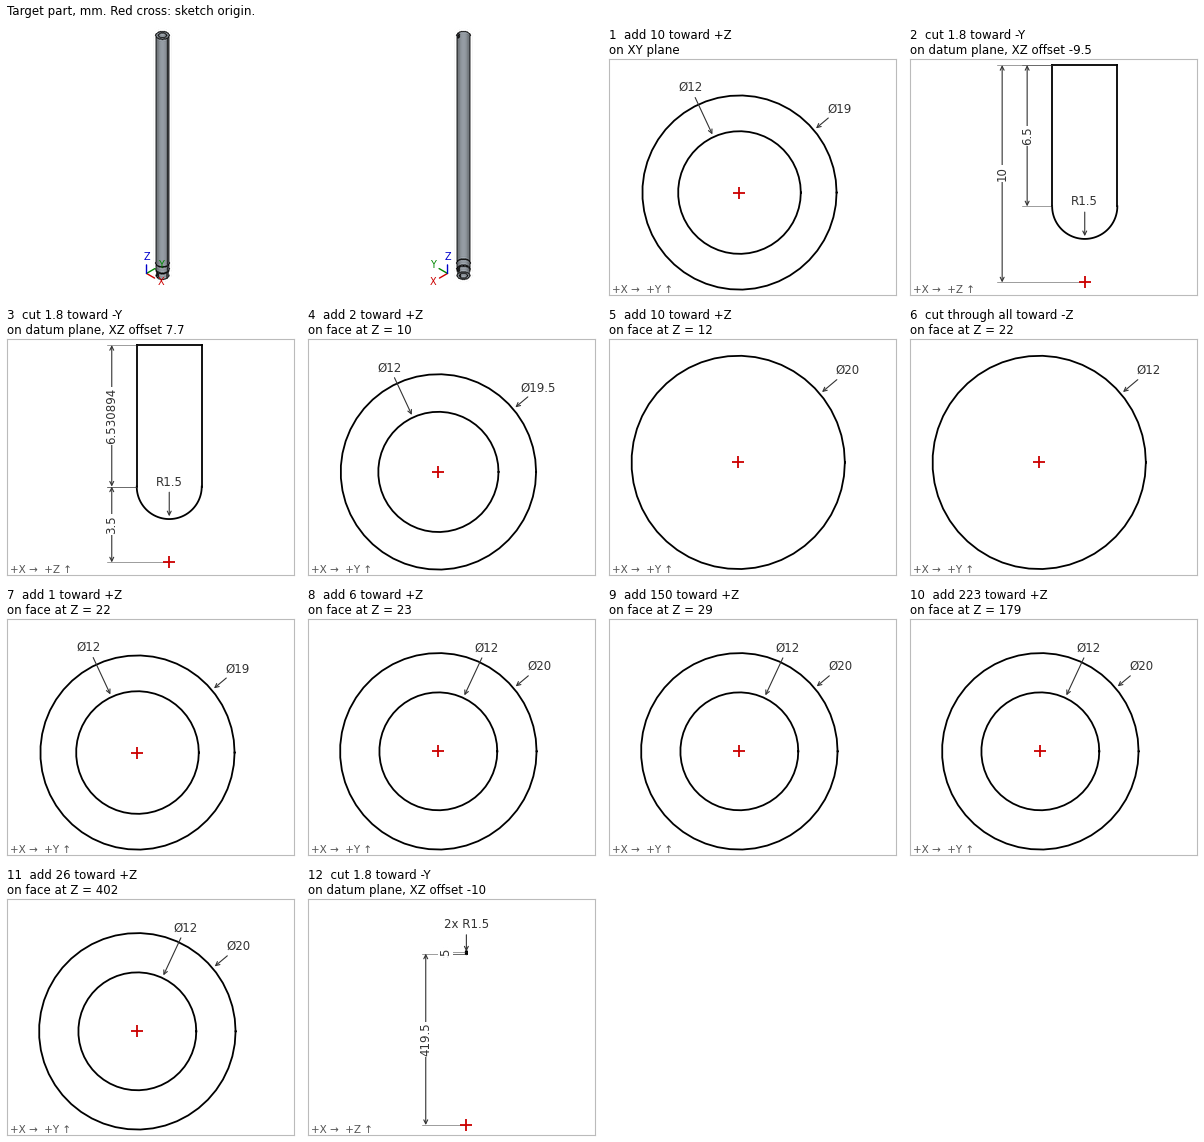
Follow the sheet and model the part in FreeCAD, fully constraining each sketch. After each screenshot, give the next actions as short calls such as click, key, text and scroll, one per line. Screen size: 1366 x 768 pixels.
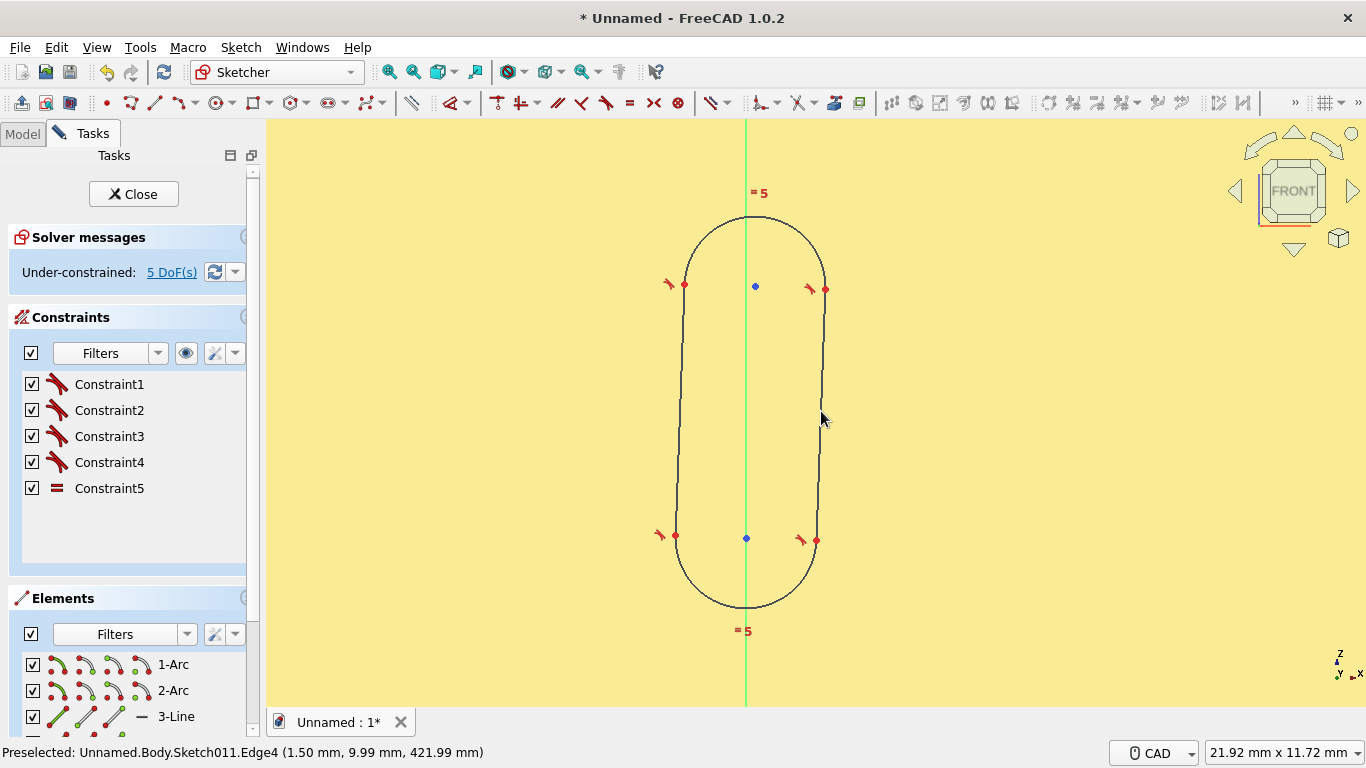
click(678, 460)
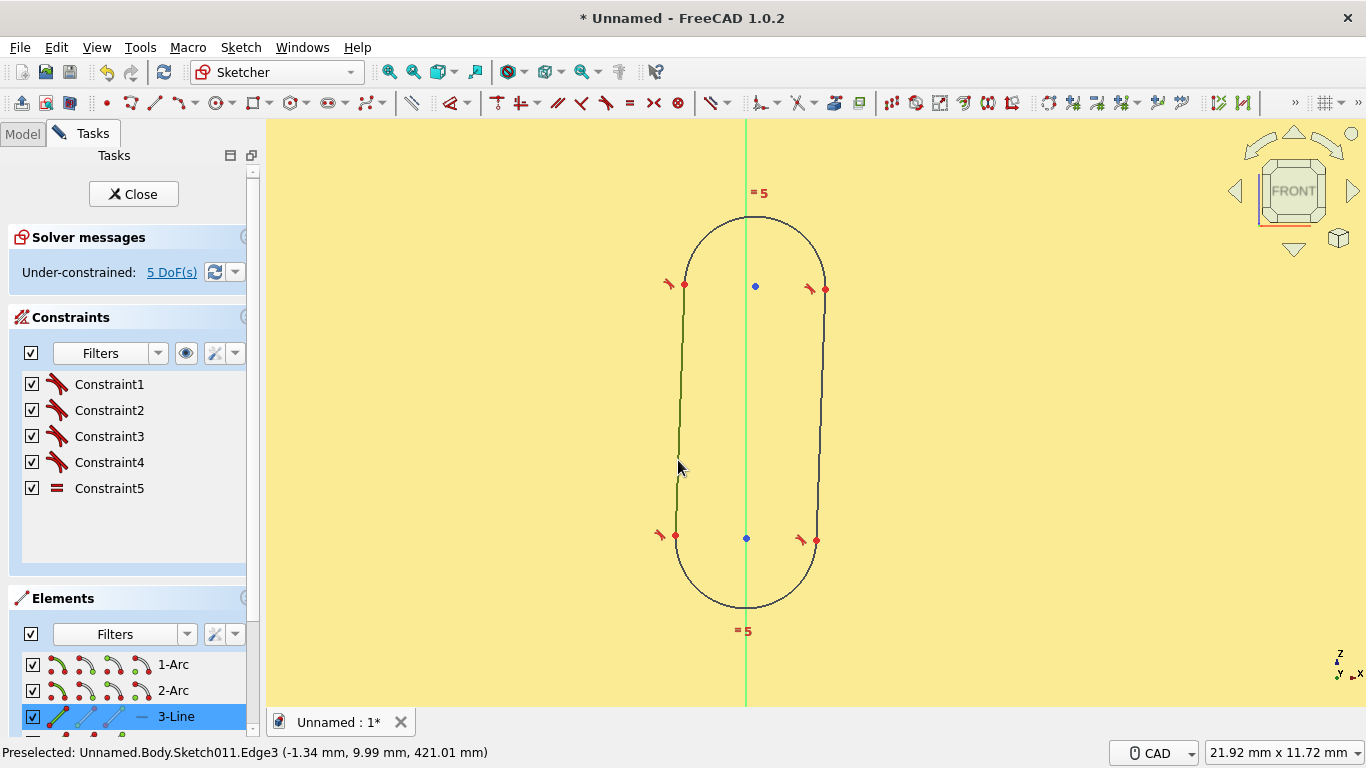
key(v)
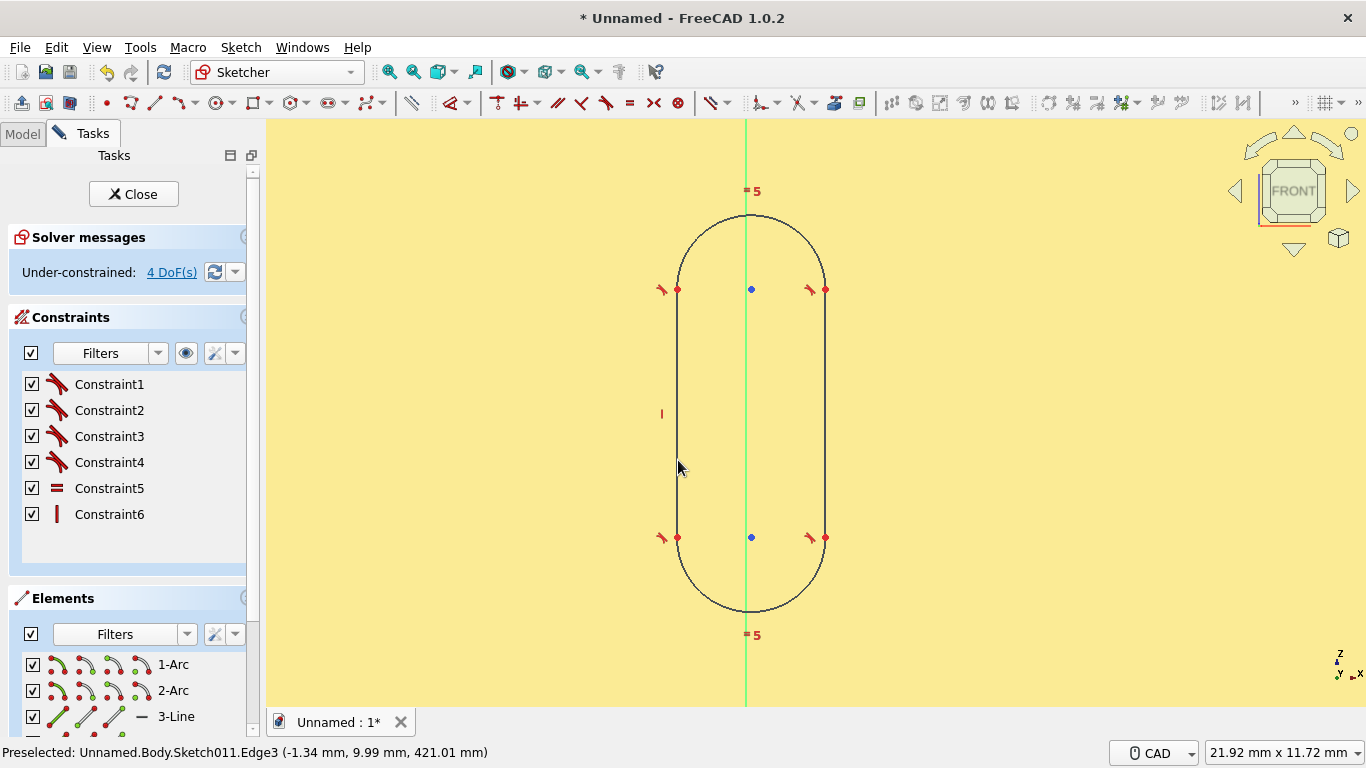
click(751, 538)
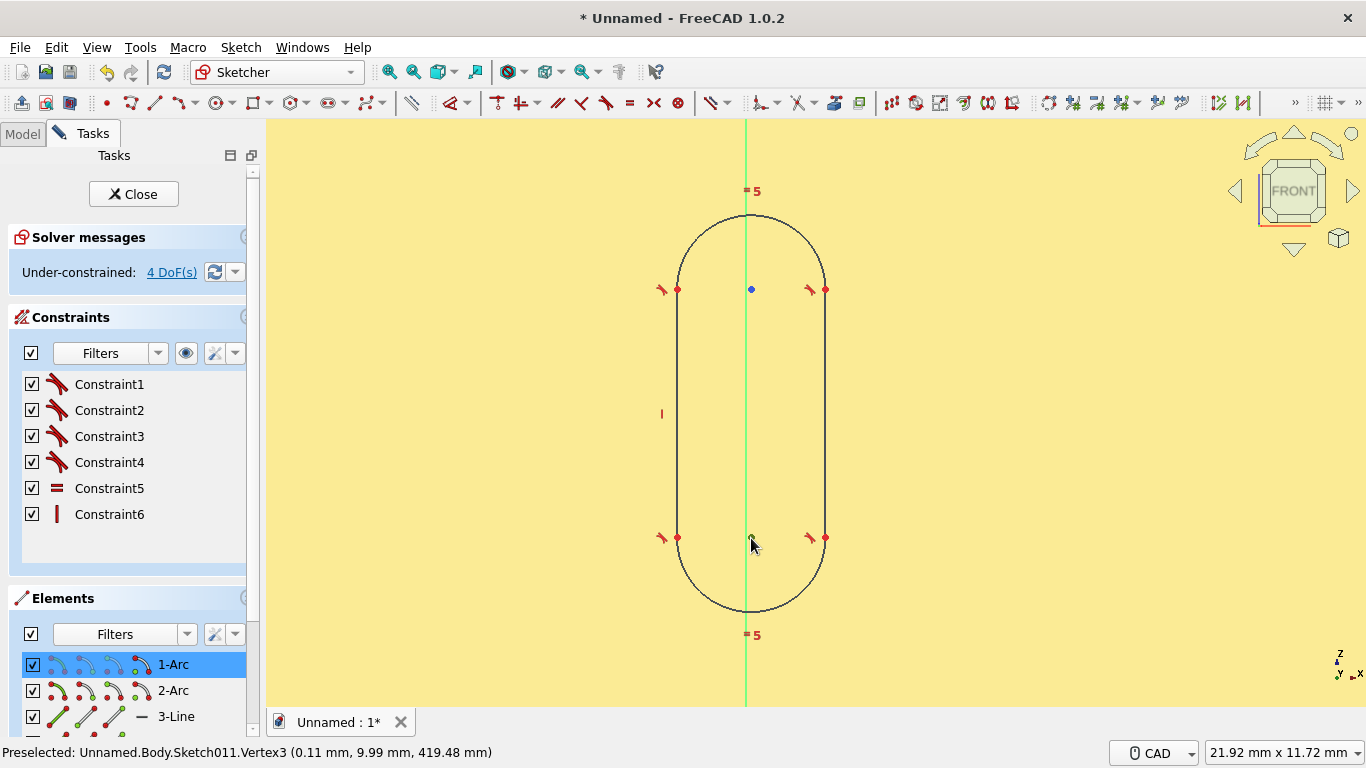
click(746, 565)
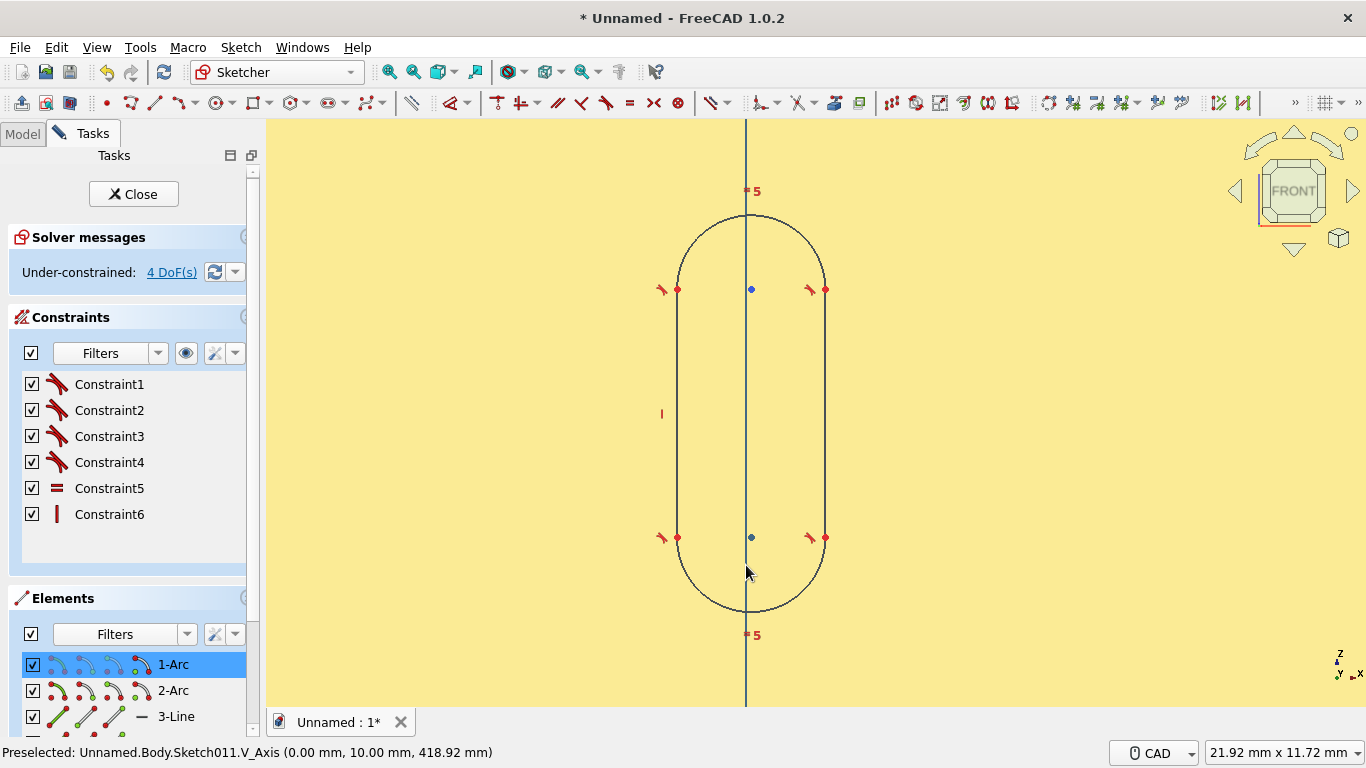
click(498, 104)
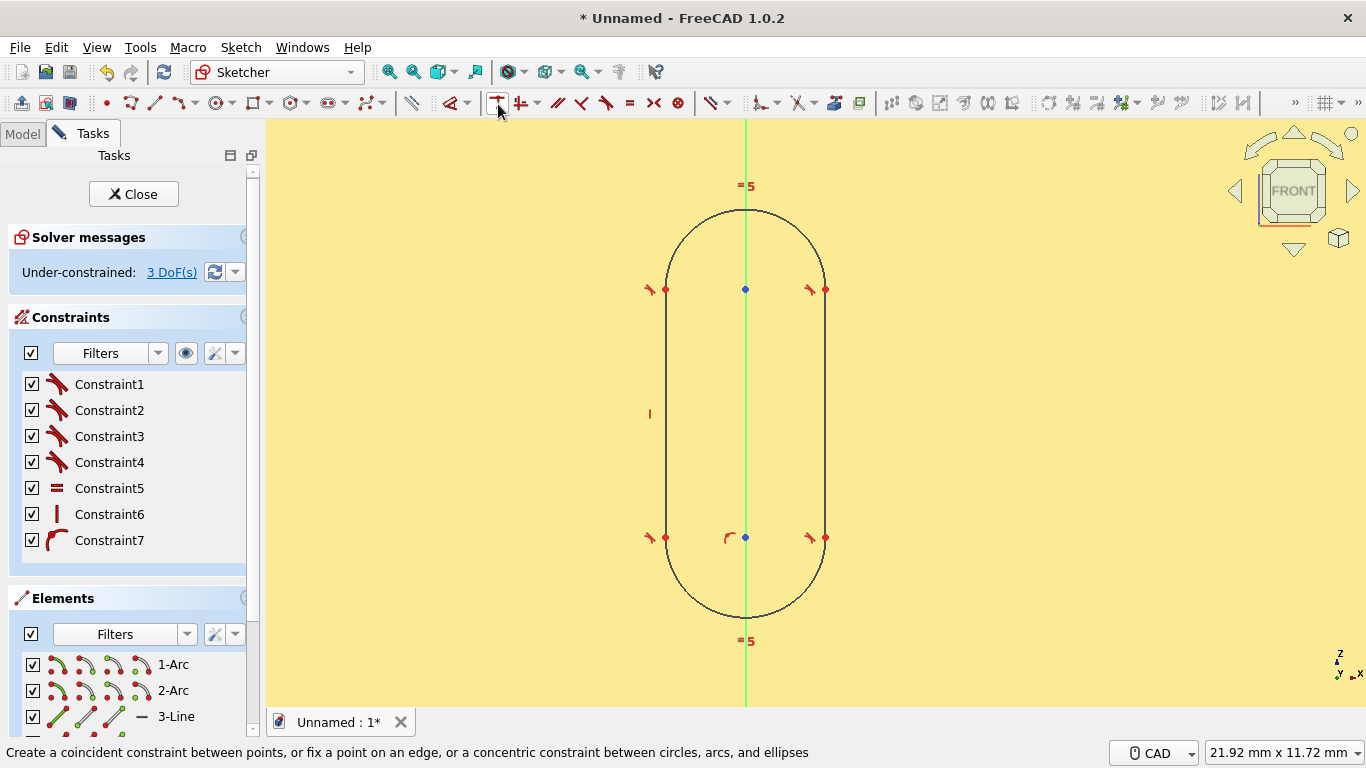
click(450, 104)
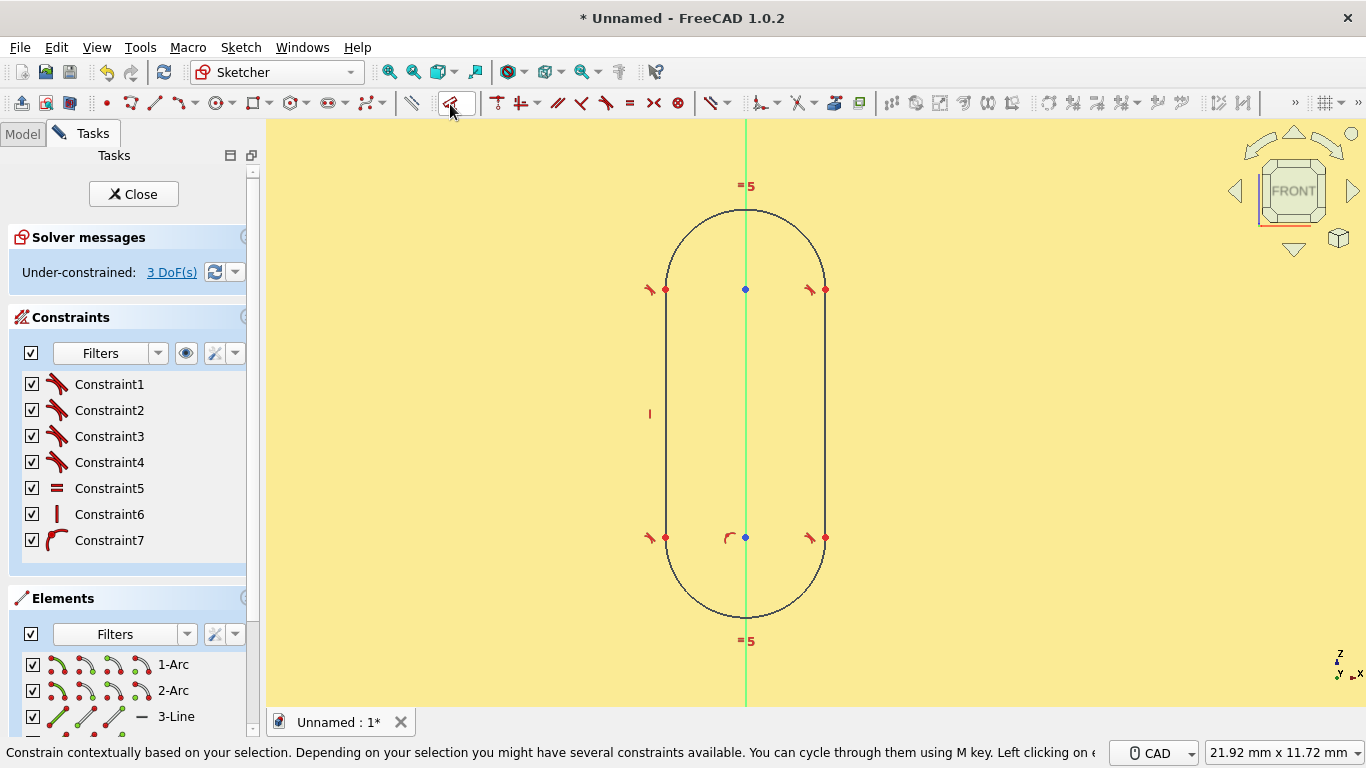
click(699, 602)
click(680, 628)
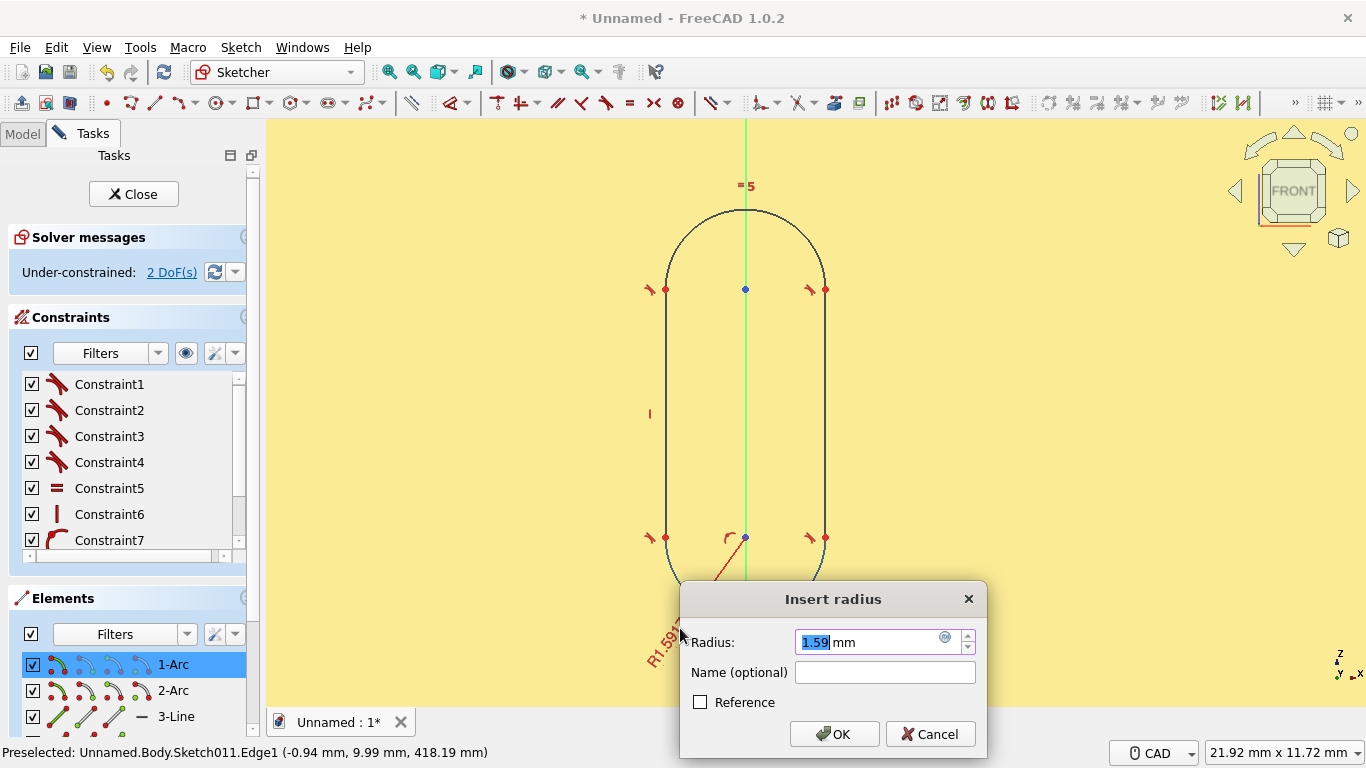
text(1.5)
key(Return)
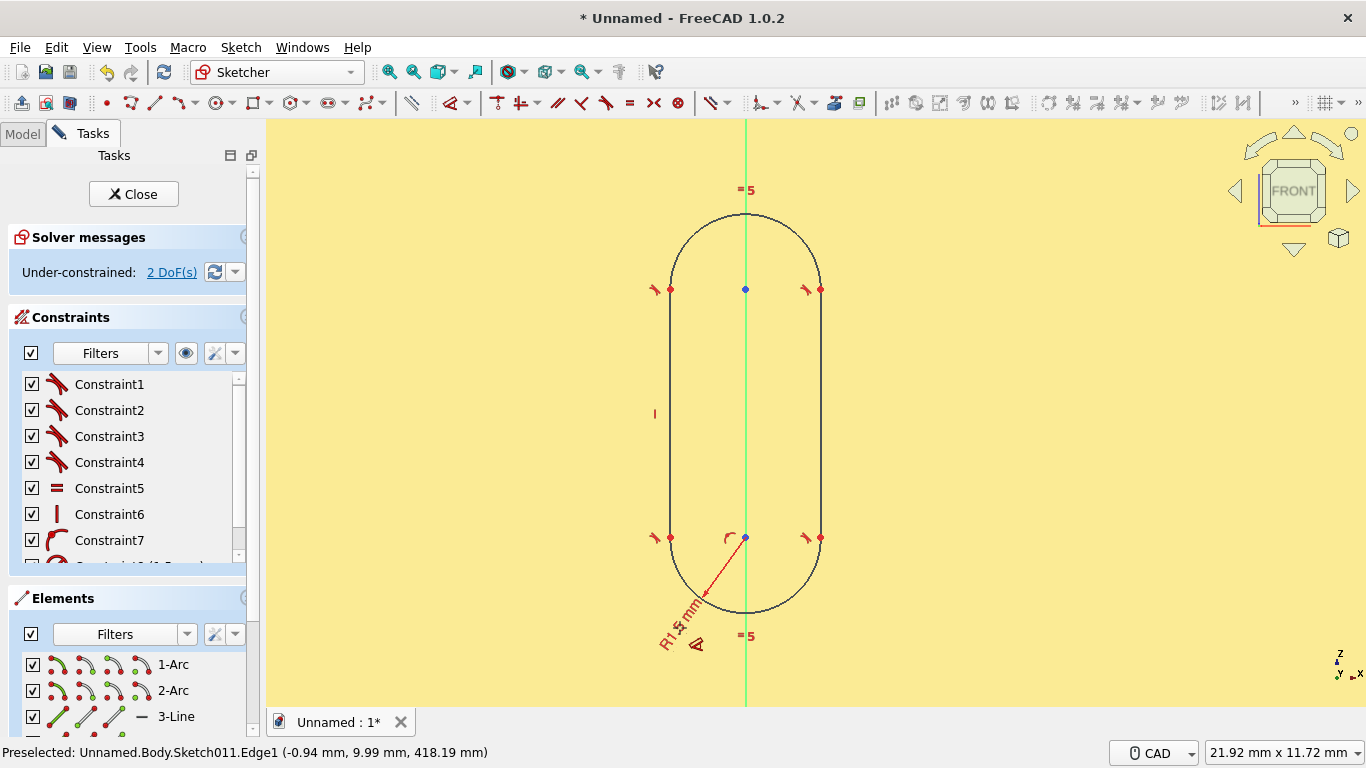
click(670, 463)
click(636, 414)